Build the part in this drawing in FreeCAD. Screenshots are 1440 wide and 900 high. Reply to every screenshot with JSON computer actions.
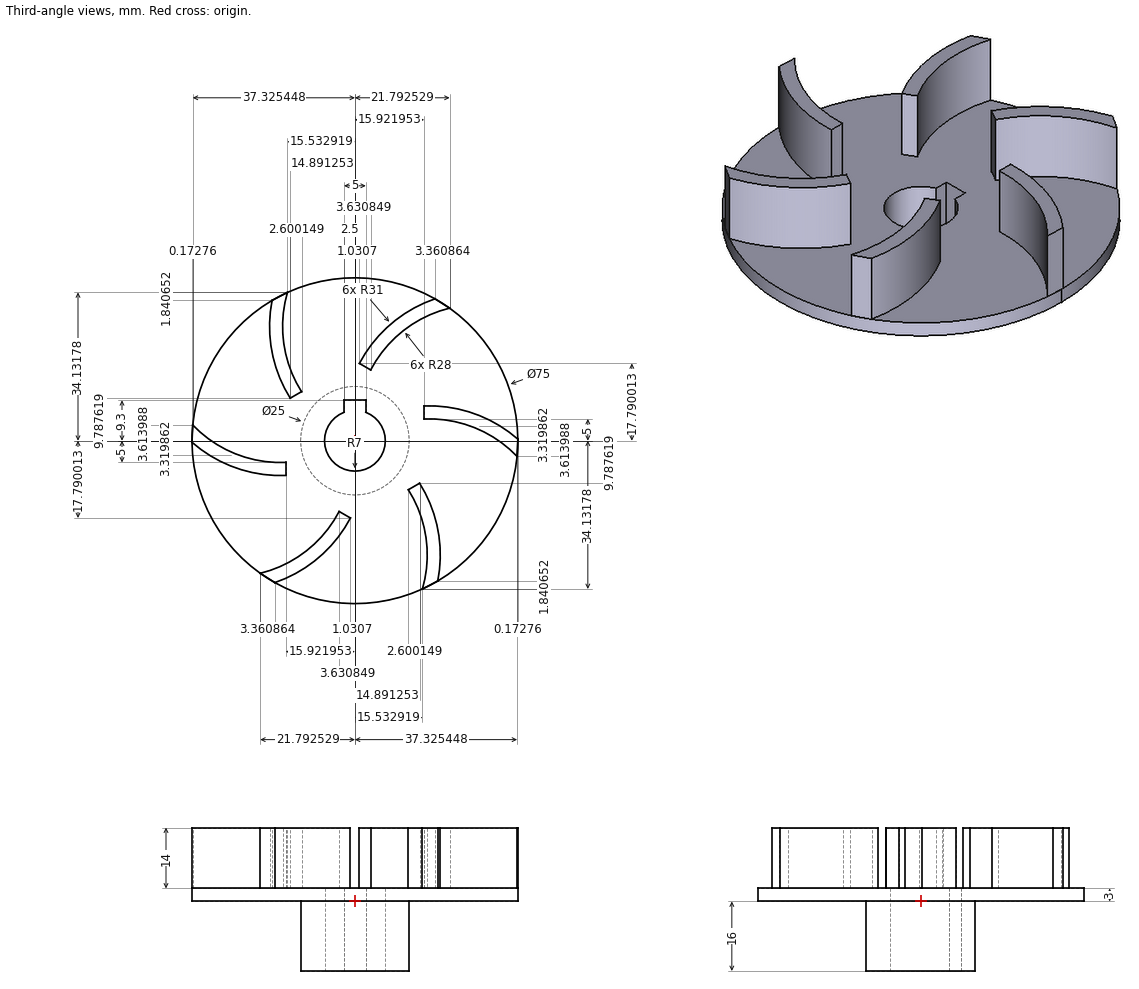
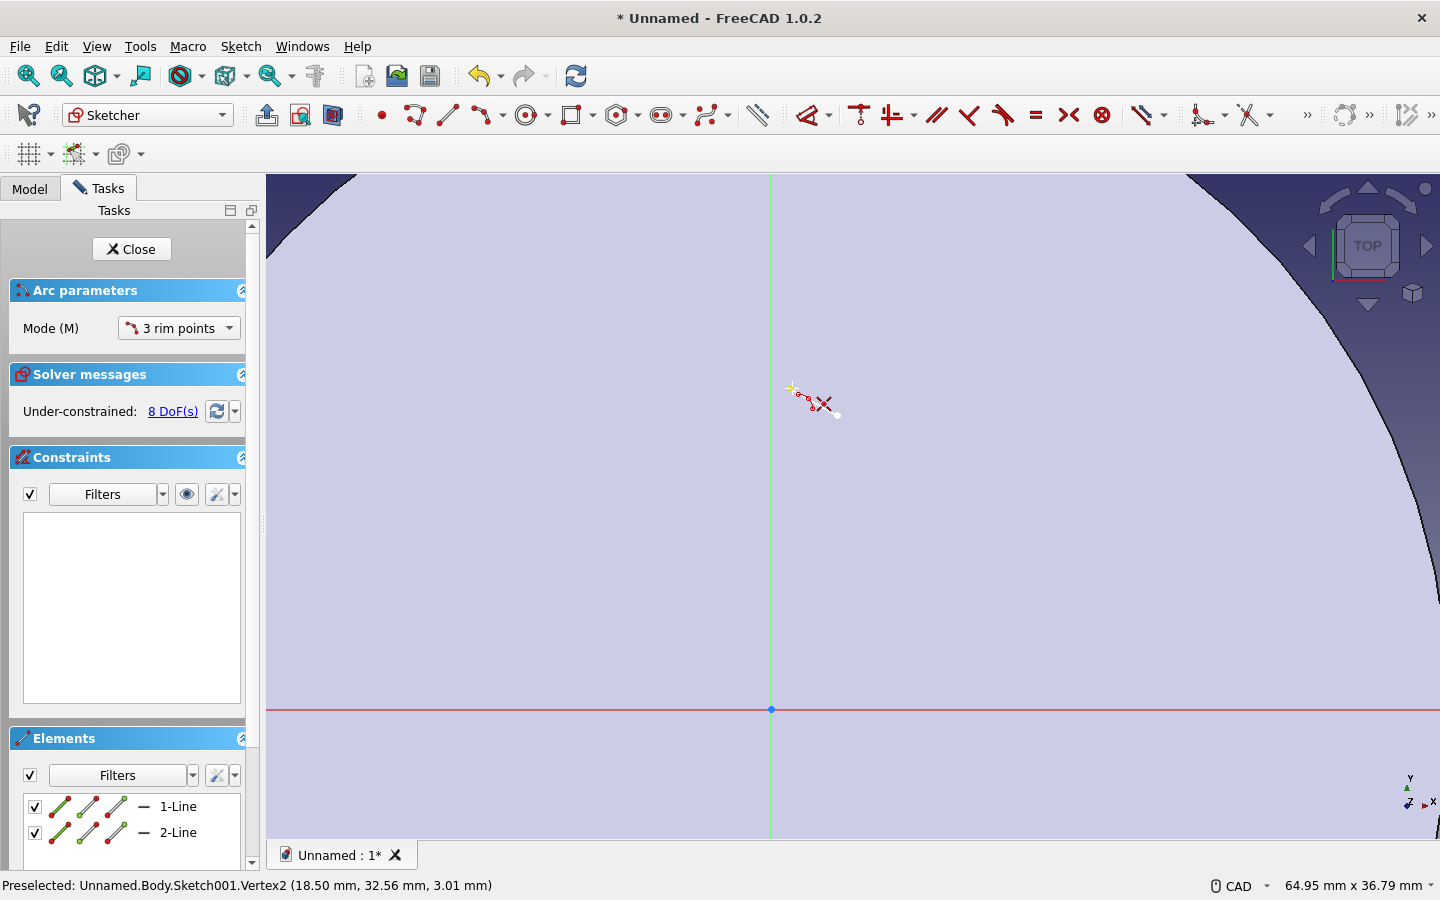
{"action": "left_click", "coordinate": [790, 389]}
{"action": "left_click", "coordinate": [922, 224]}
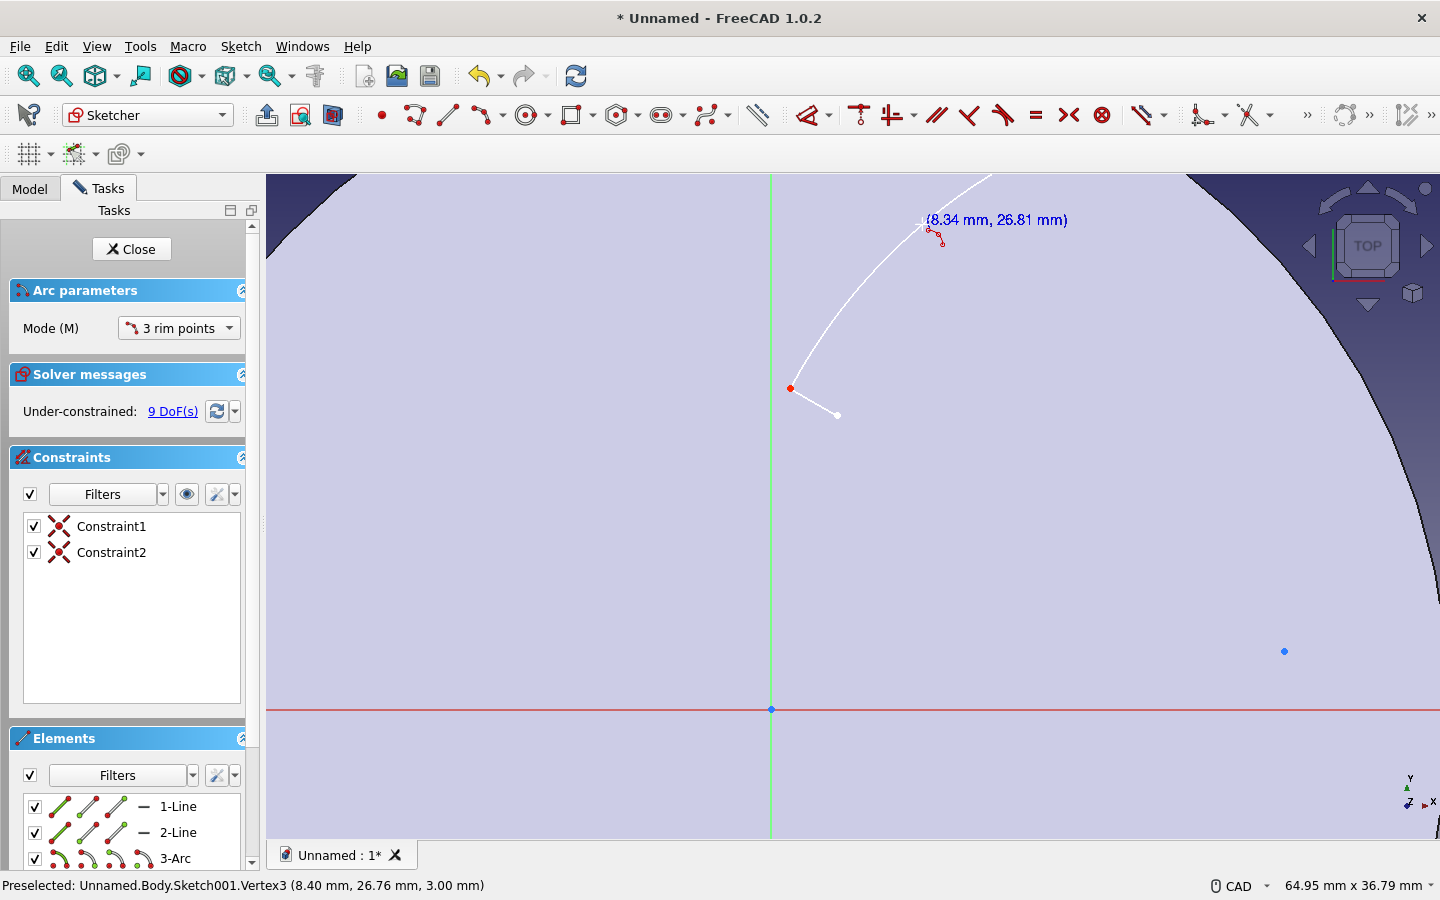
{"action": "left_click", "coordinate": [837, 416]}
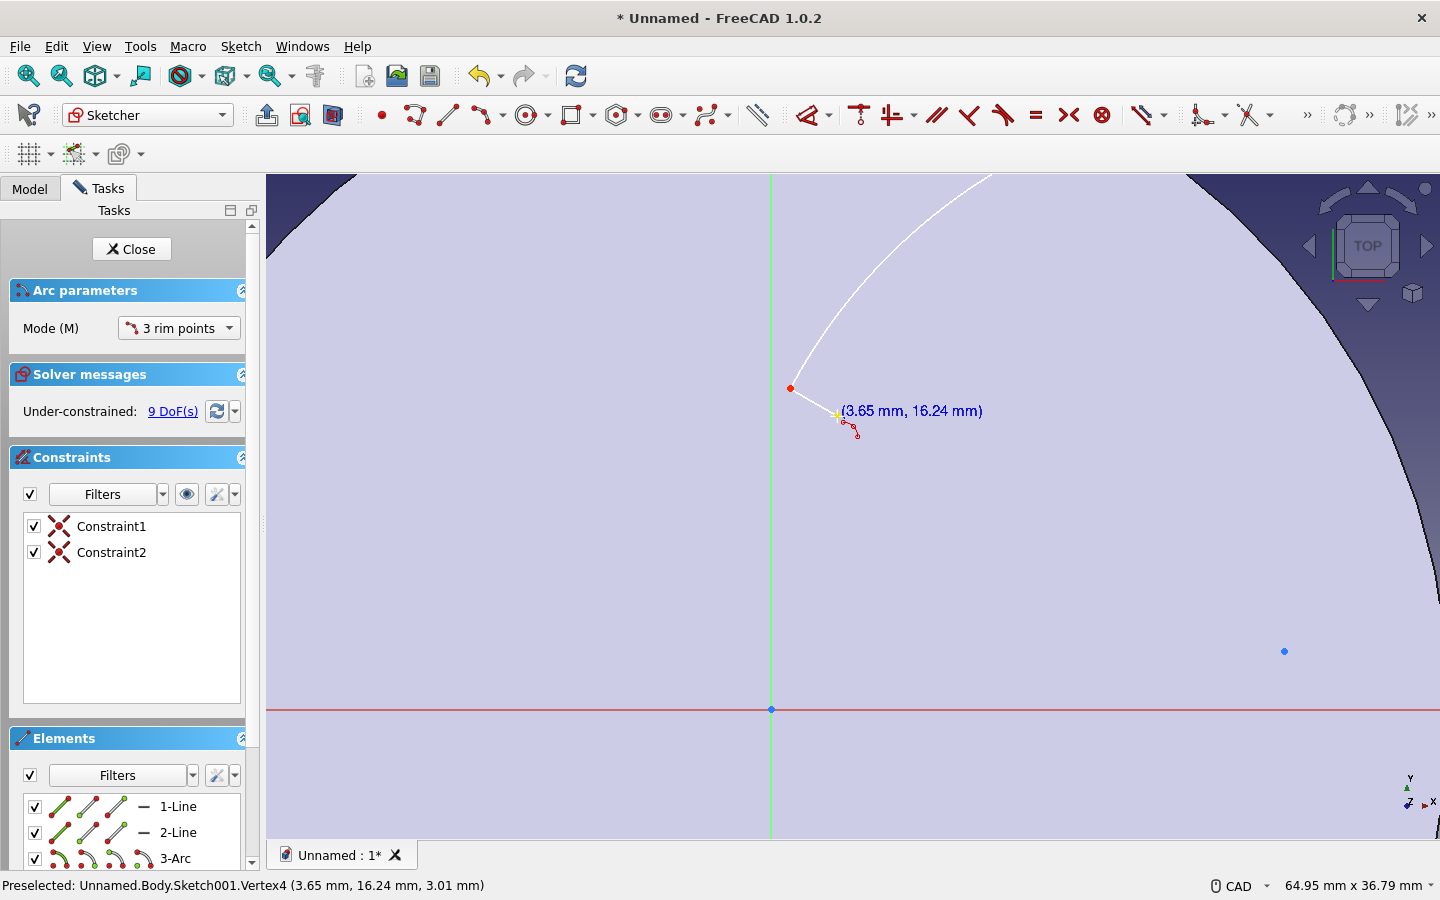
{"action": "scroll", "coordinate": [792, 388], "scroll_direction": "down", "scroll_amount": 5}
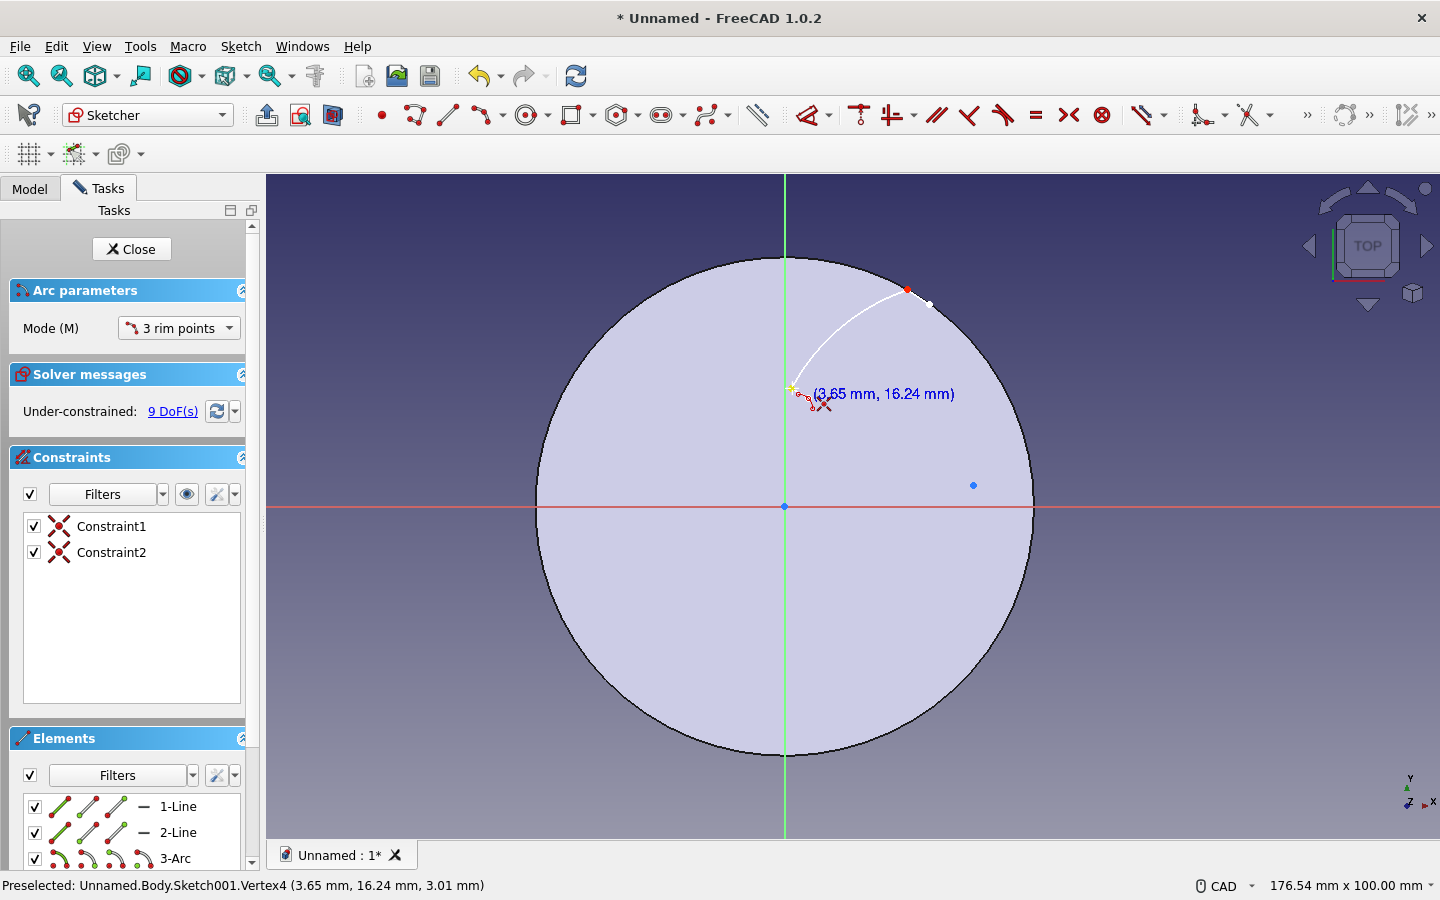
{"action": "left_click", "coordinate": [930, 305]}
{"action": "left_click", "coordinate": [859, 338]}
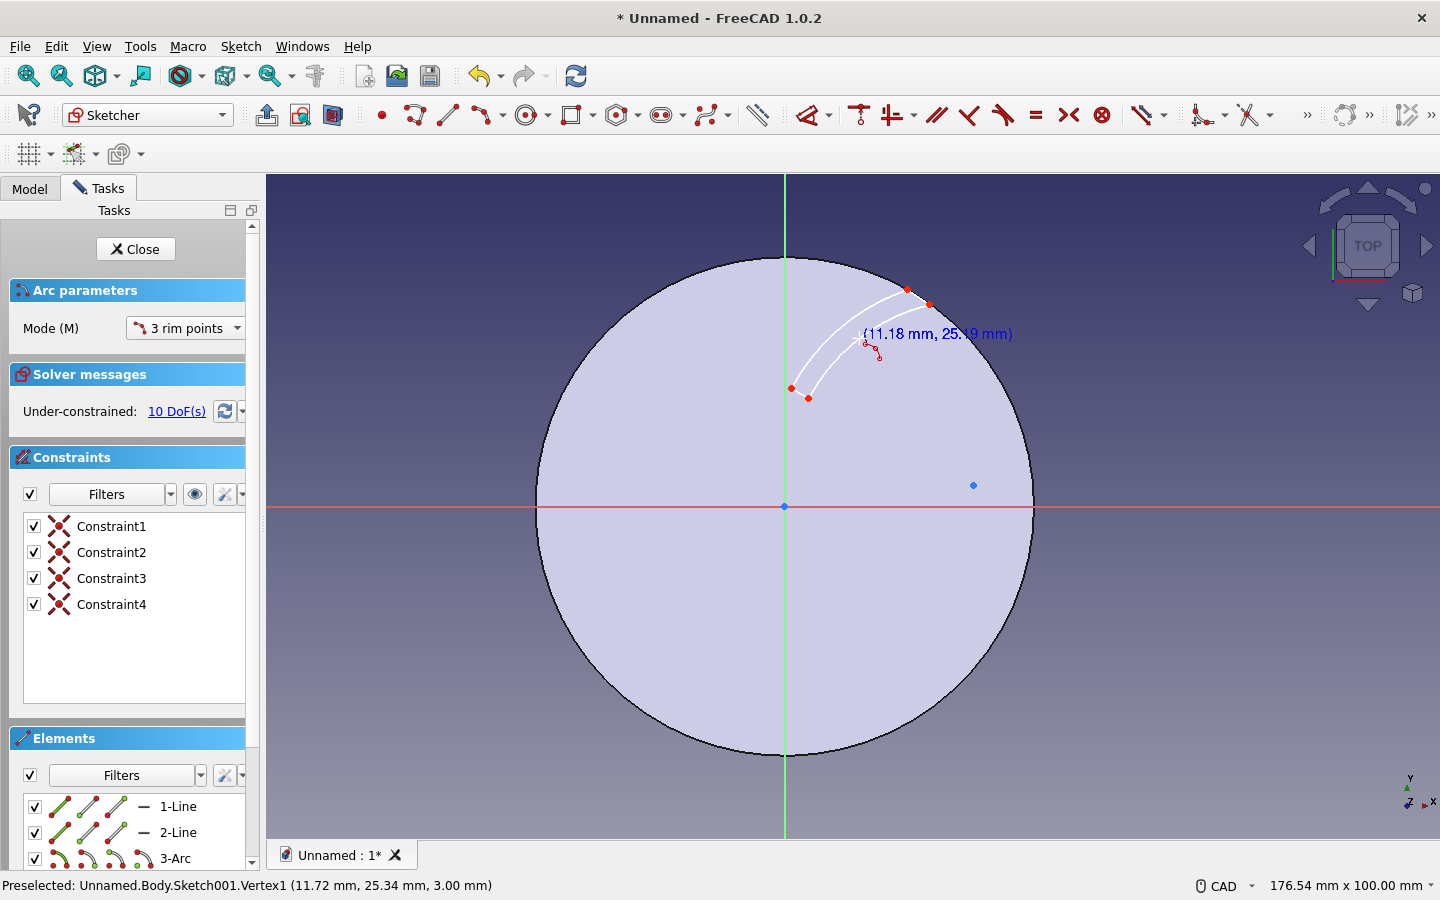
{"action": "left_click", "coordinate": [448, 116]}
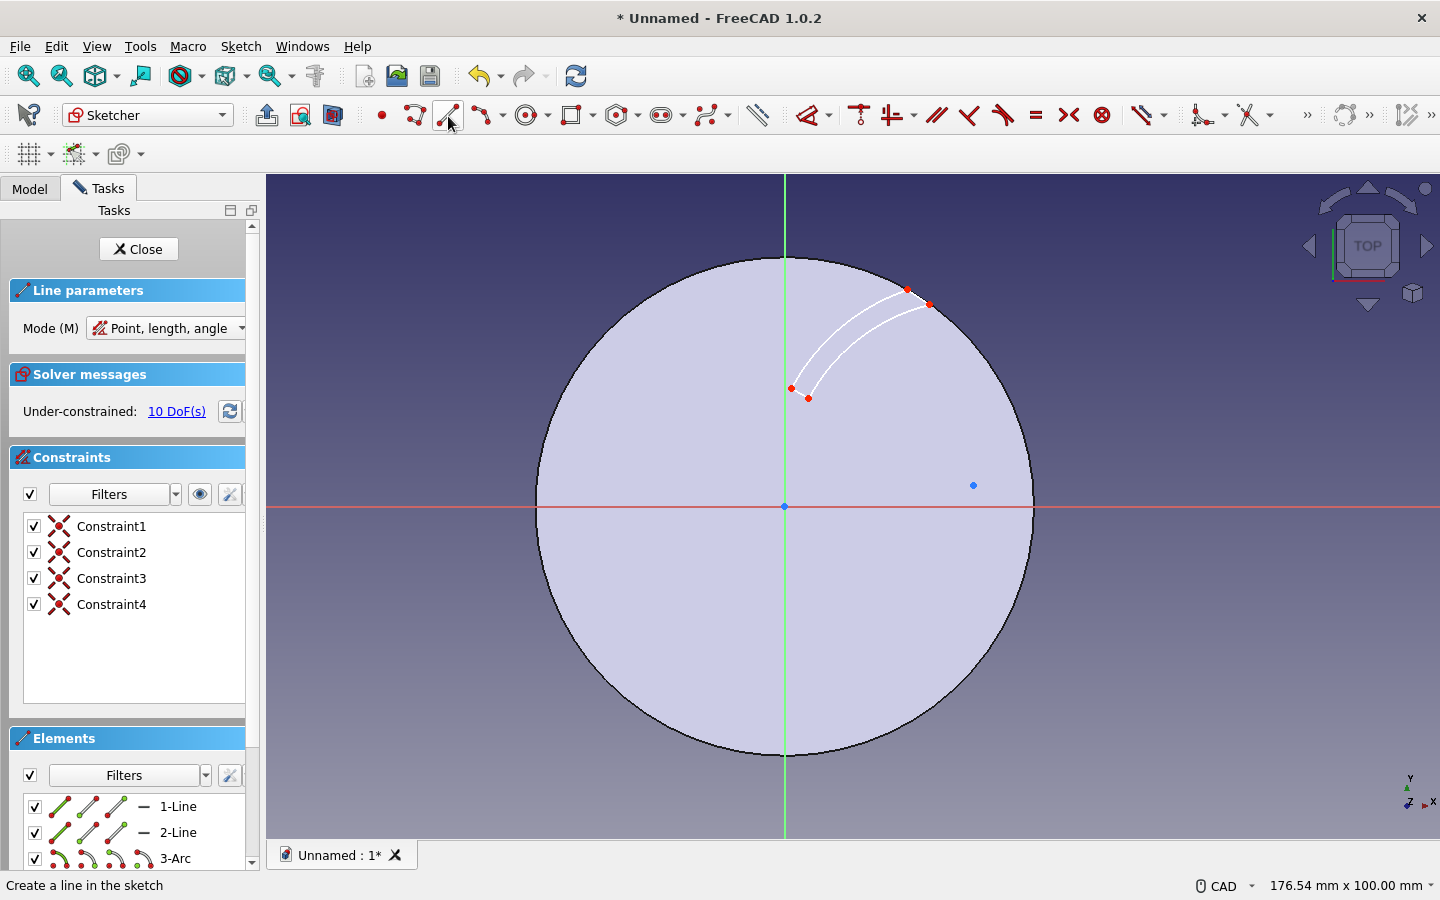
{"action": "left_click", "coordinate": [681, 280]}
{"action": "left_click", "coordinate": [658, 292]}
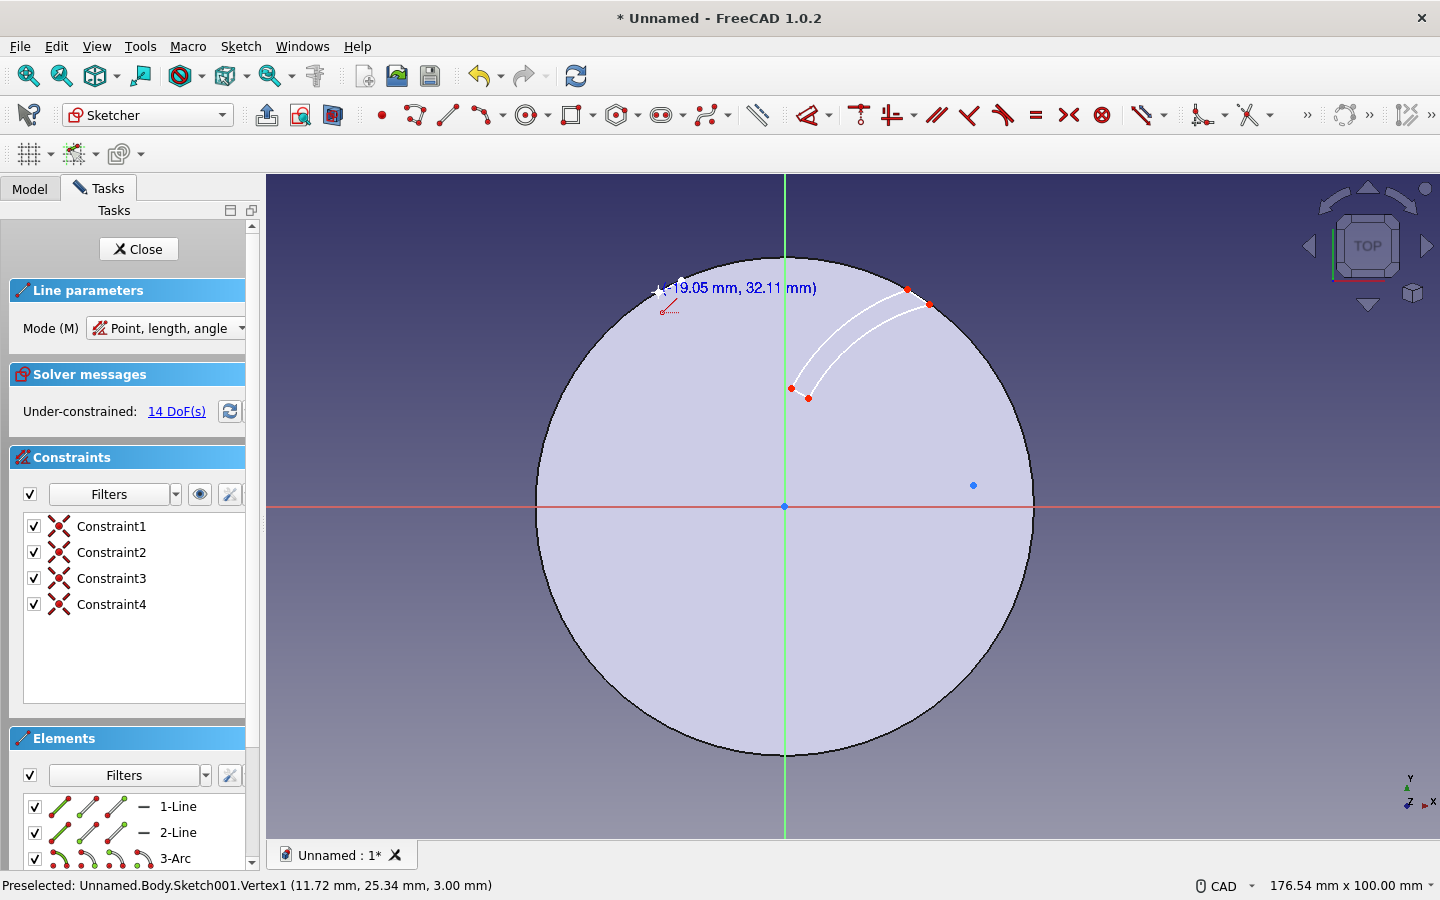
{"action": "left_click", "coordinate": [686, 441]}
{"action": "left_click", "coordinate": [703, 431]}